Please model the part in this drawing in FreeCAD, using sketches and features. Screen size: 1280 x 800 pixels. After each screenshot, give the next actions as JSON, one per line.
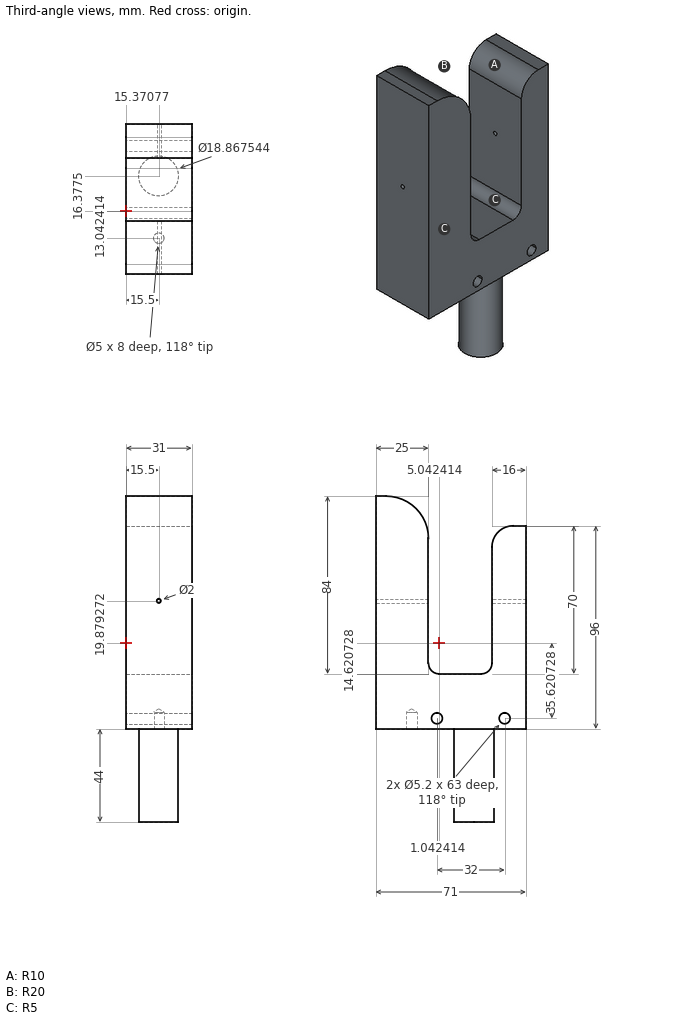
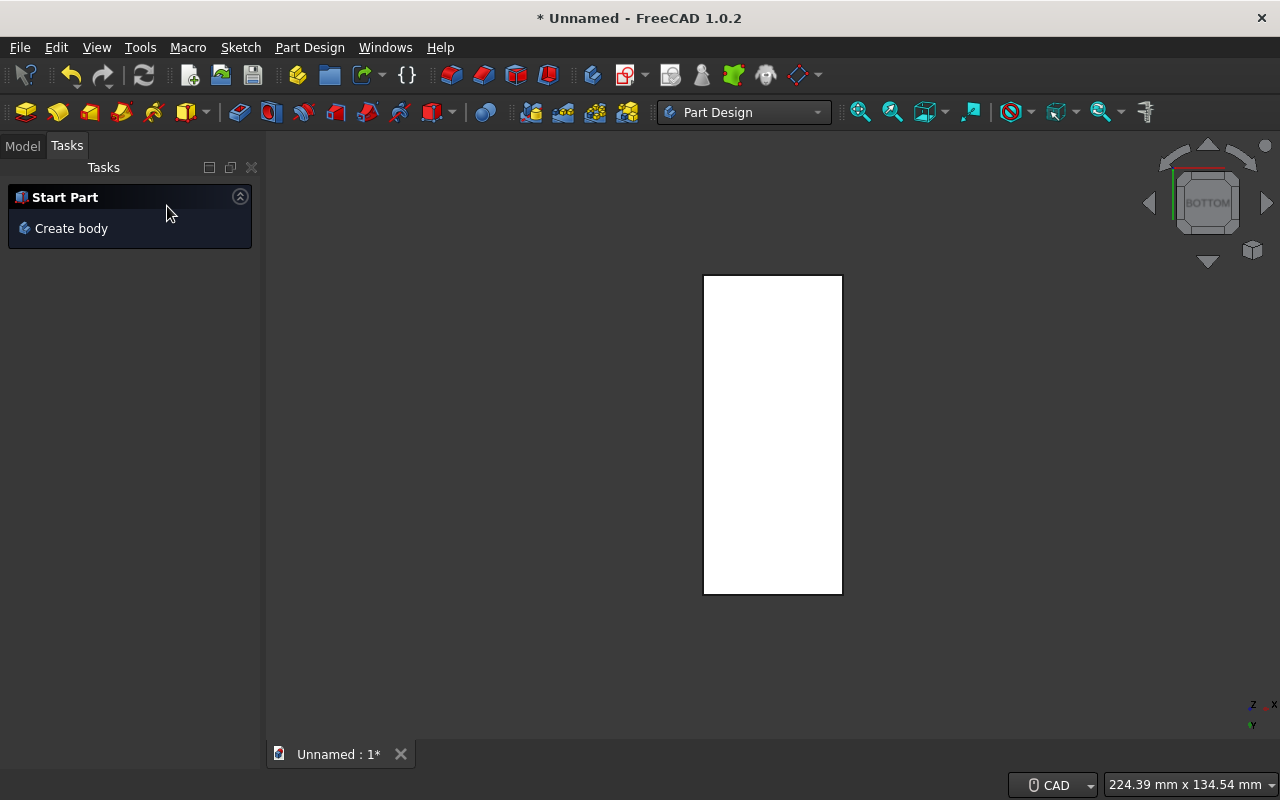
{"action": "left_click", "coordinate": [773, 480]}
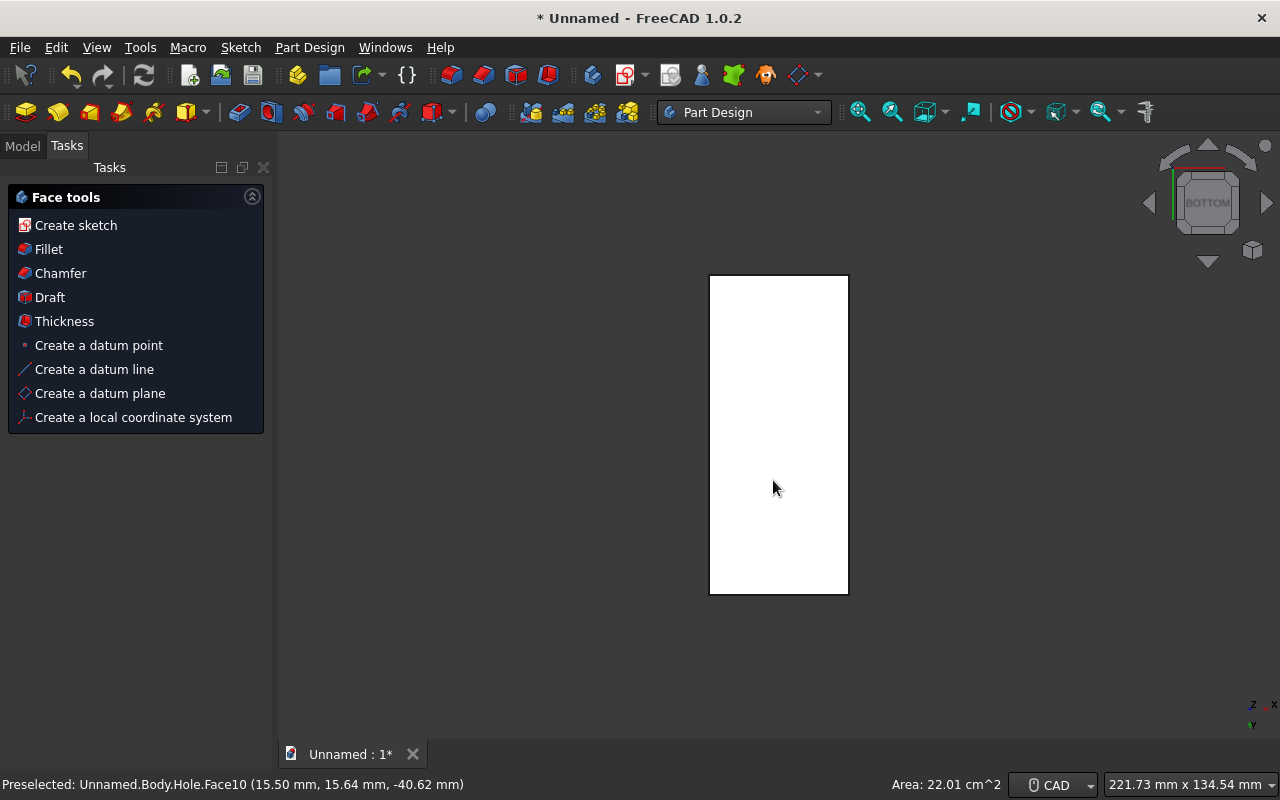
{"action": "left_click", "coordinate": [626, 76]}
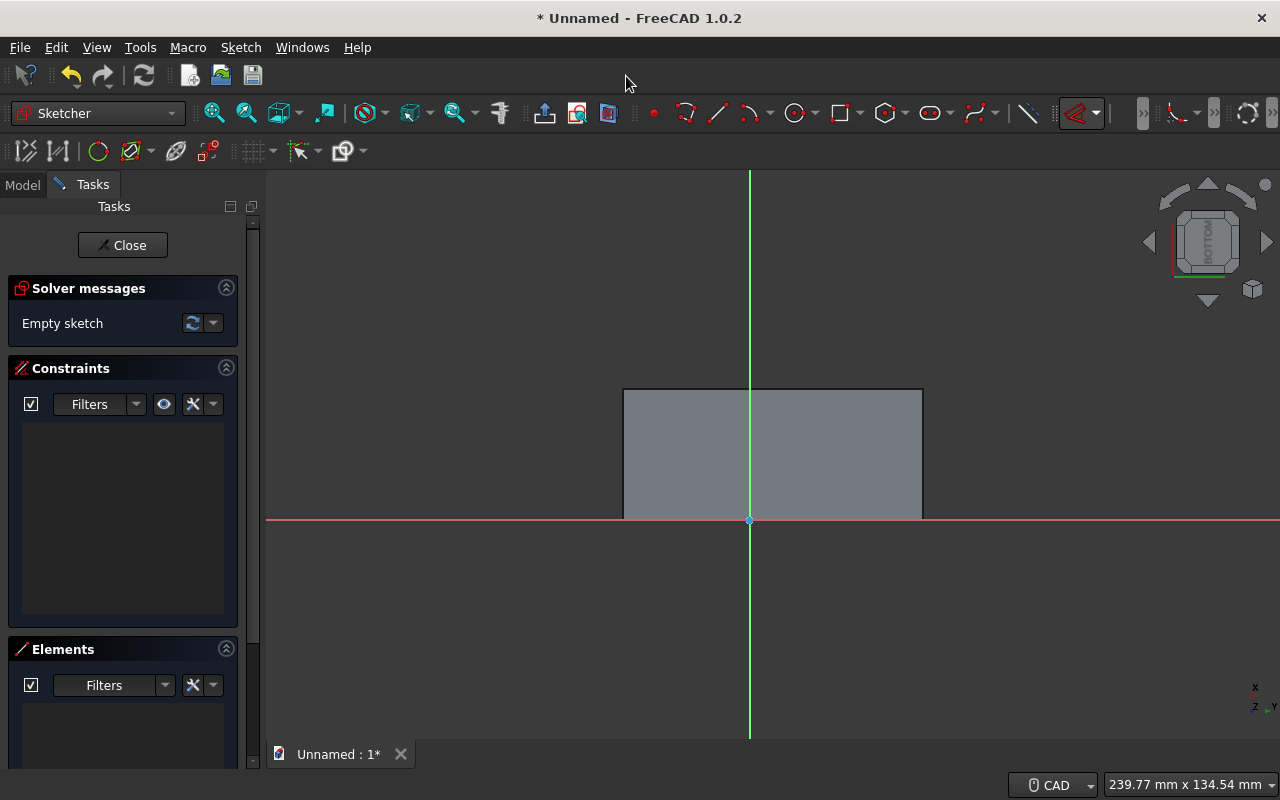
{"action": "scroll", "coordinate": [694, 455], "scroll_direction": "up", "scroll_amount": 14}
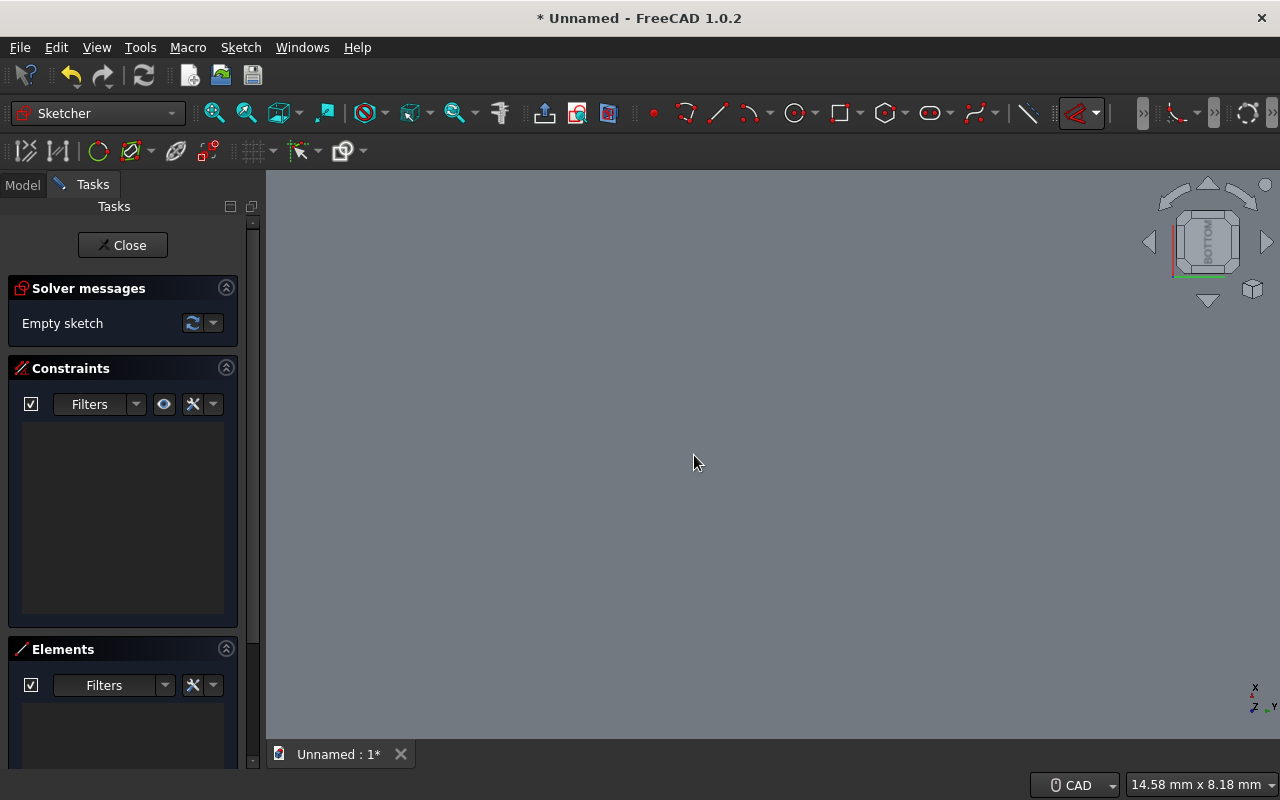
{"action": "left_click", "coordinate": [796, 114]}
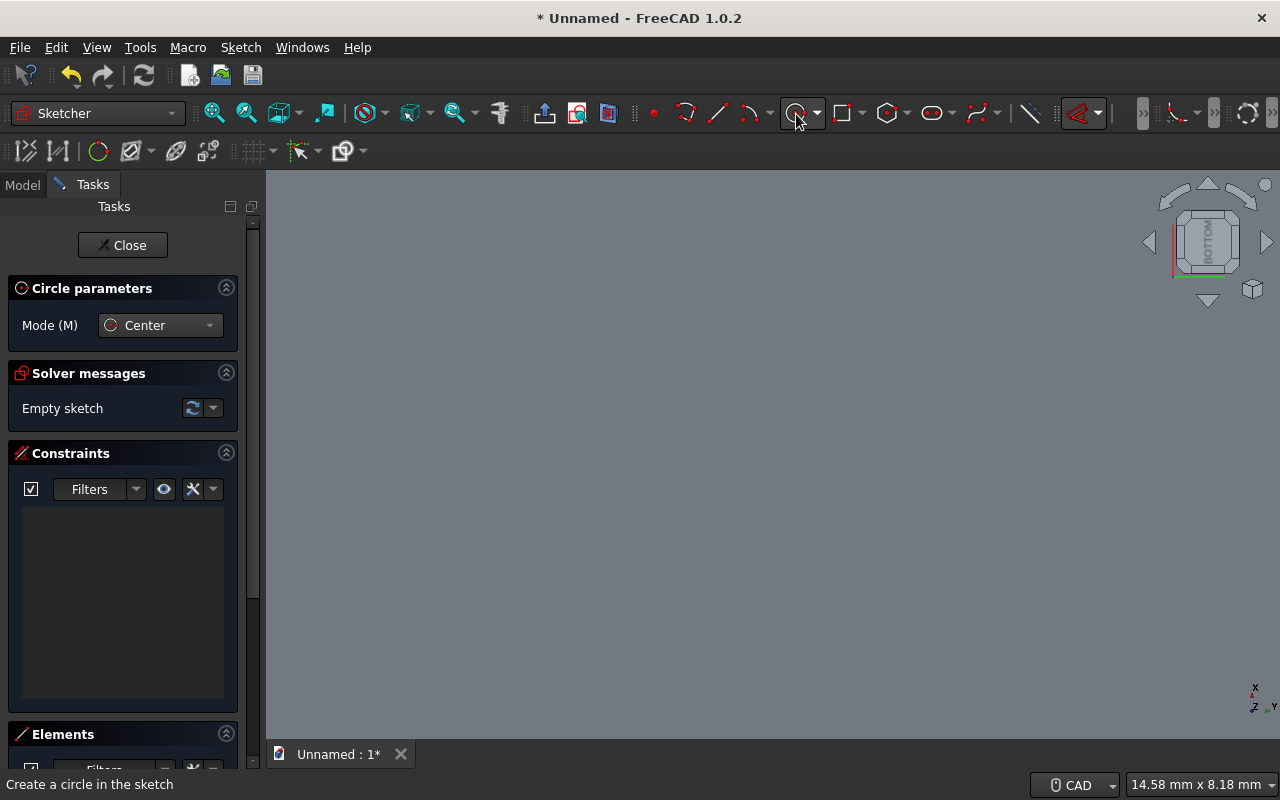
{"action": "left_click", "coordinate": [700, 439]}
{"action": "mouse_move", "coordinate": [823, 316]}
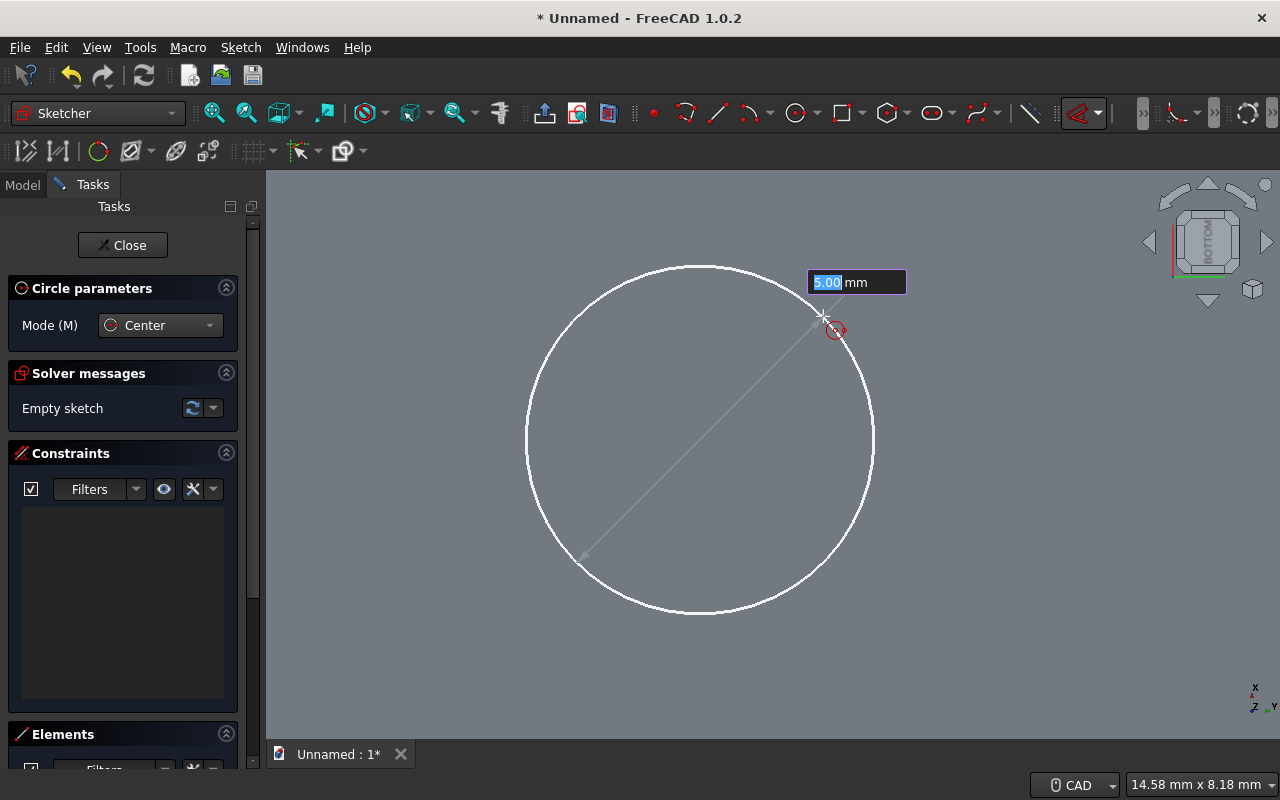
{"action": "type", "text": "5"}
{"action": "key", "text": "Return"}
{"action": "key", "text": "Escape"}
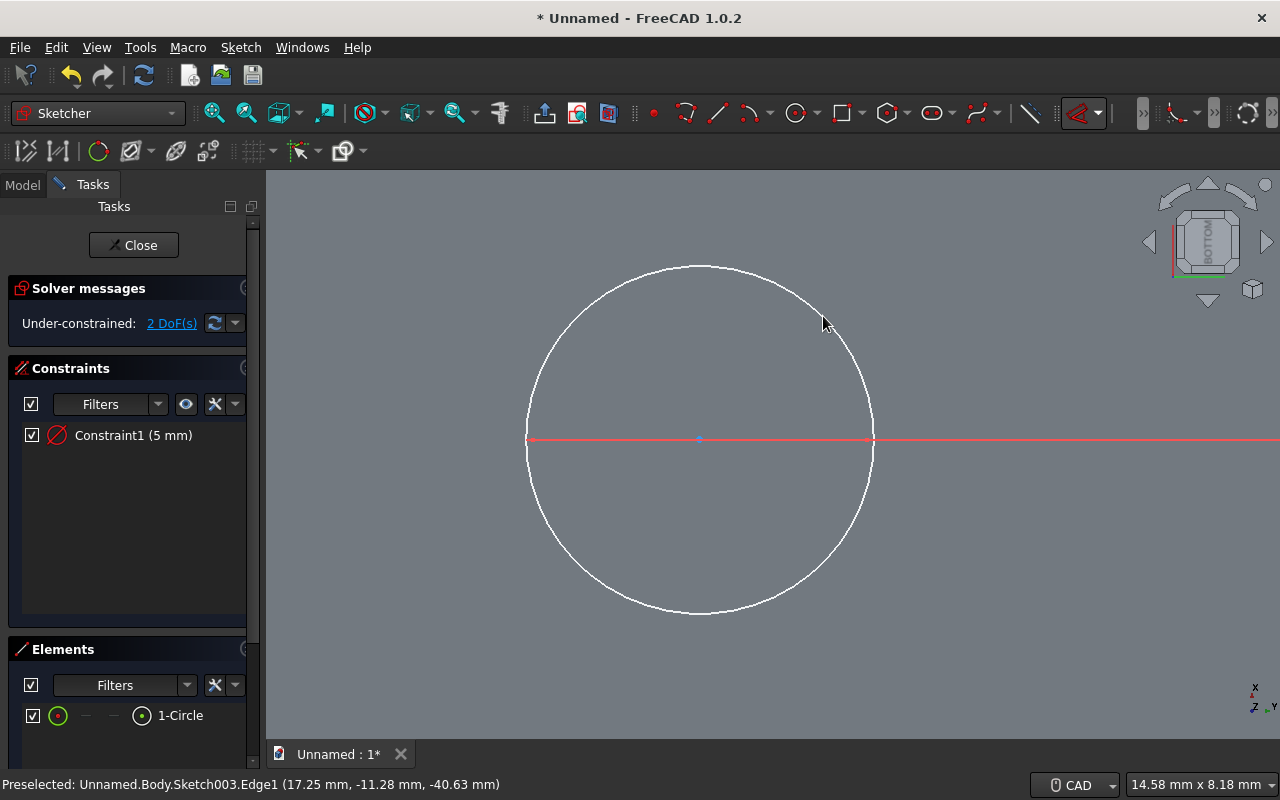
{"action": "left_click", "coordinate": [700, 440]}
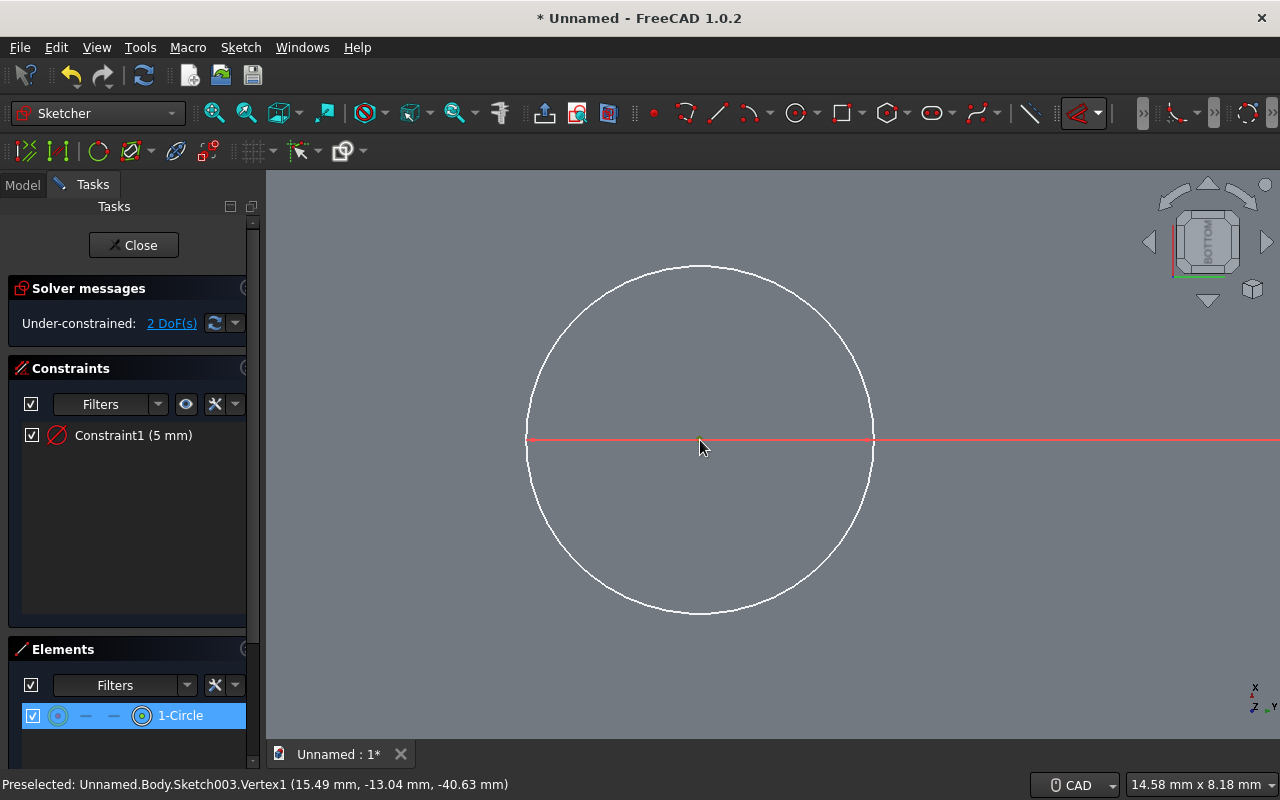
{"action": "left_click", "coordinate": [1100, 114]}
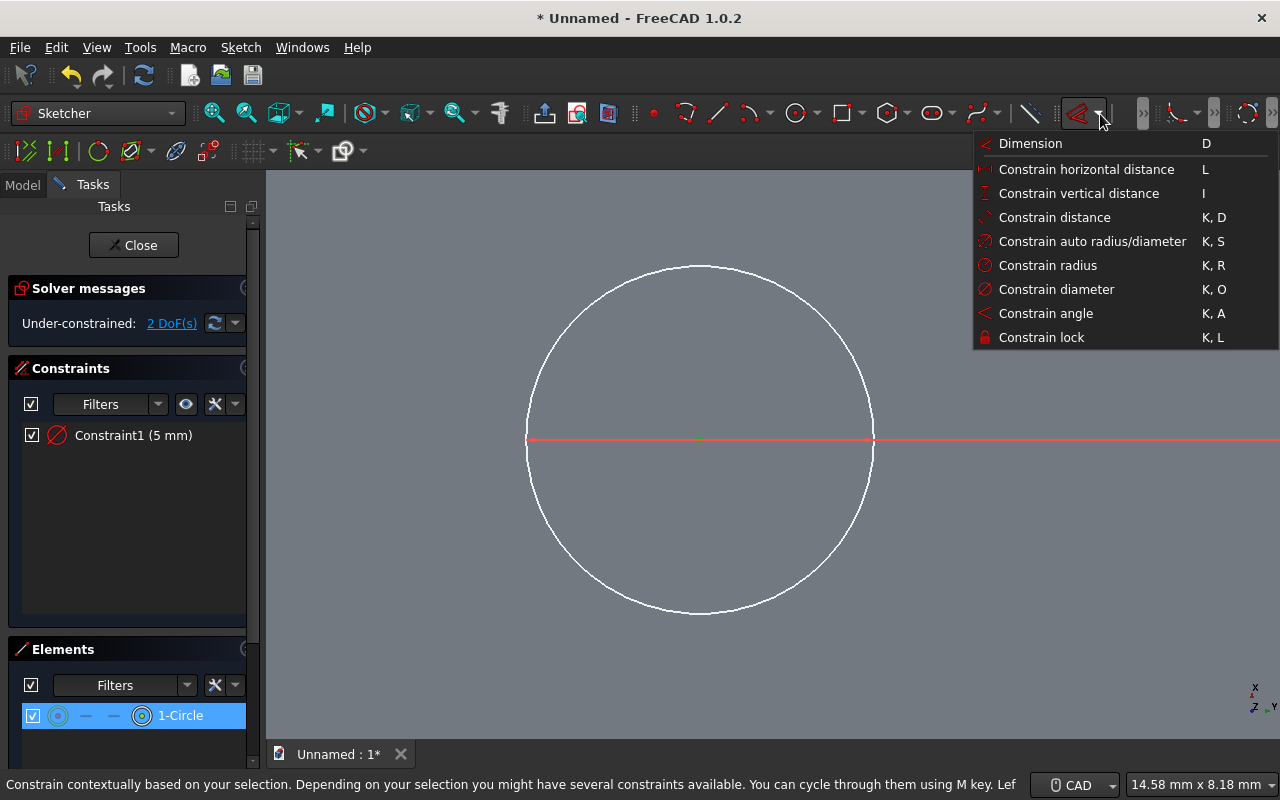
{"action": "left_click", "coordinate": [1126, 193]}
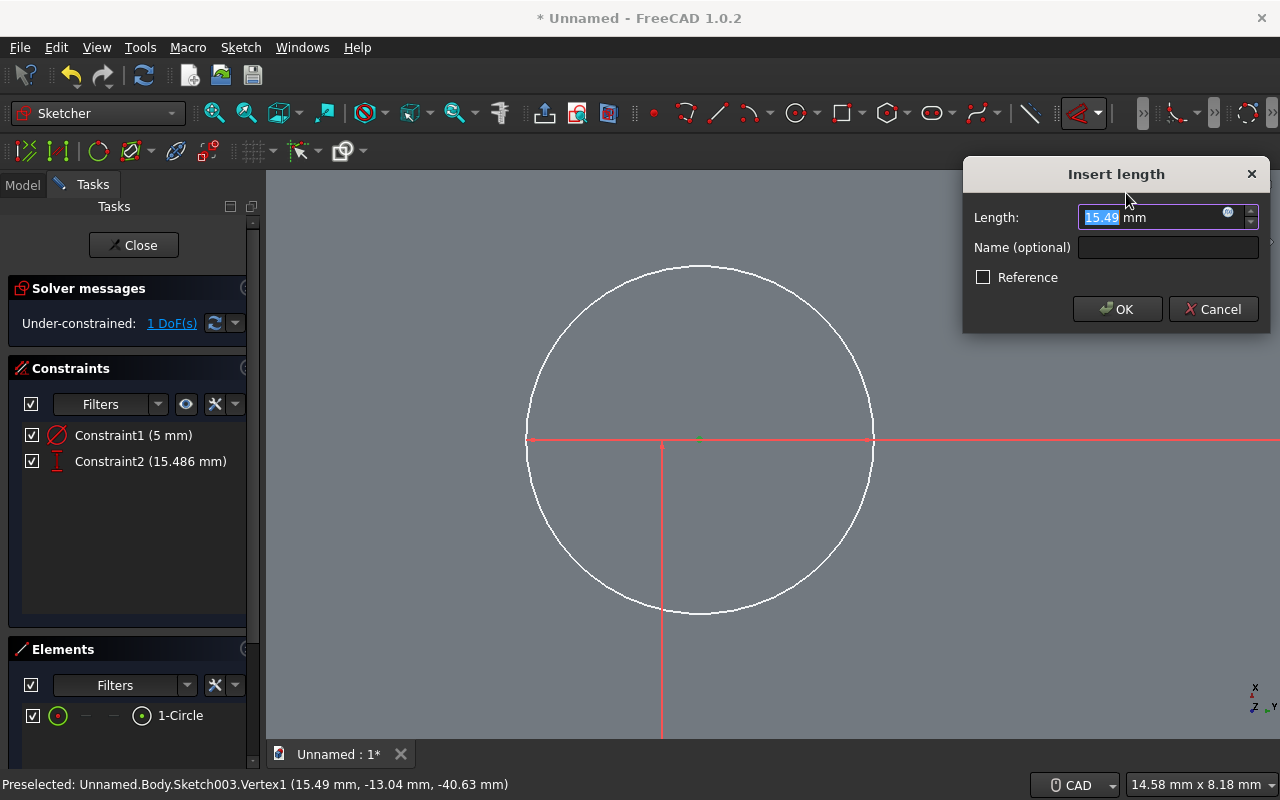
{"action": "type", "text": "15.5"}
{"action": "key", "text": "Return"}